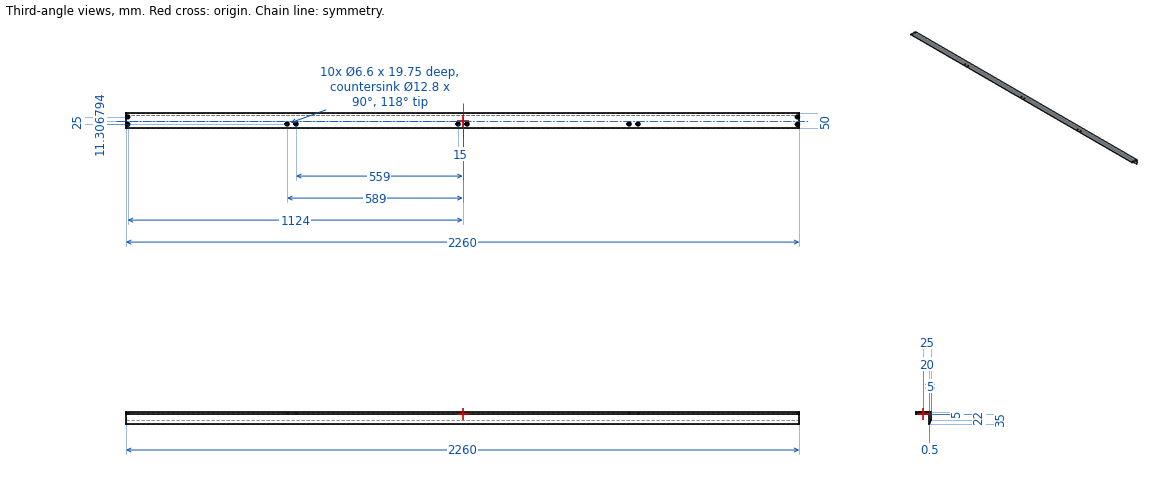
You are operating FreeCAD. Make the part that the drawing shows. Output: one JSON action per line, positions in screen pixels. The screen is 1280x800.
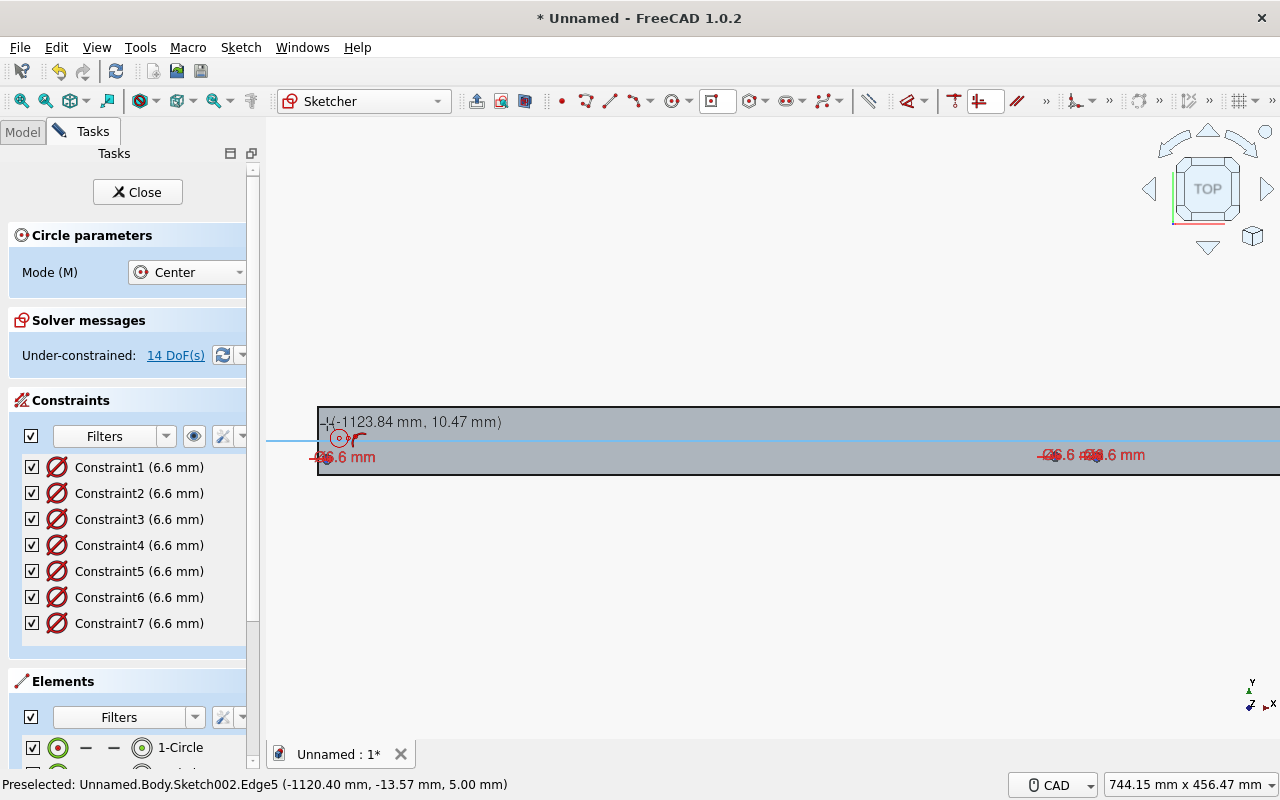
{"action": "left_click", "coordinate": [327, 424]}
{"action": "mouse_move", "coordinate": [330, 421]}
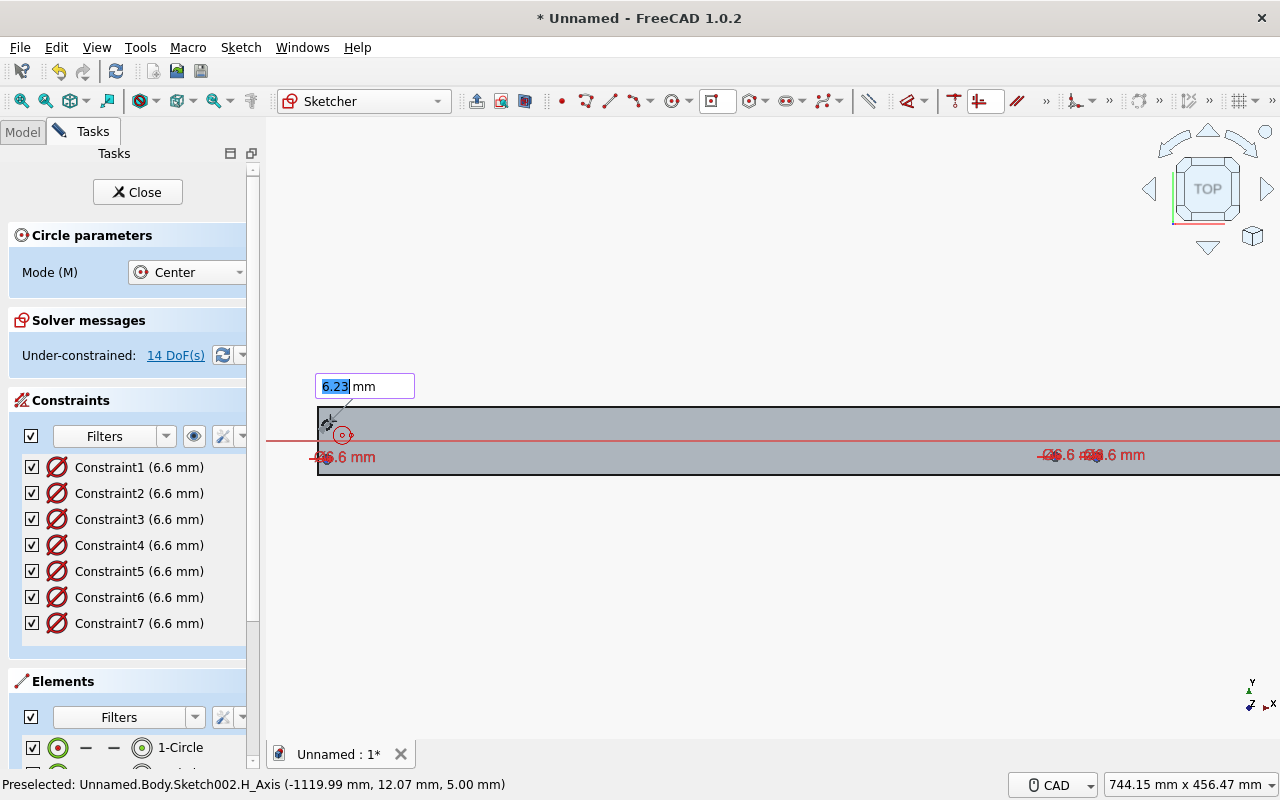
{"action": "type", "text": "6.6"}
{"action": "key", "text": "Return"}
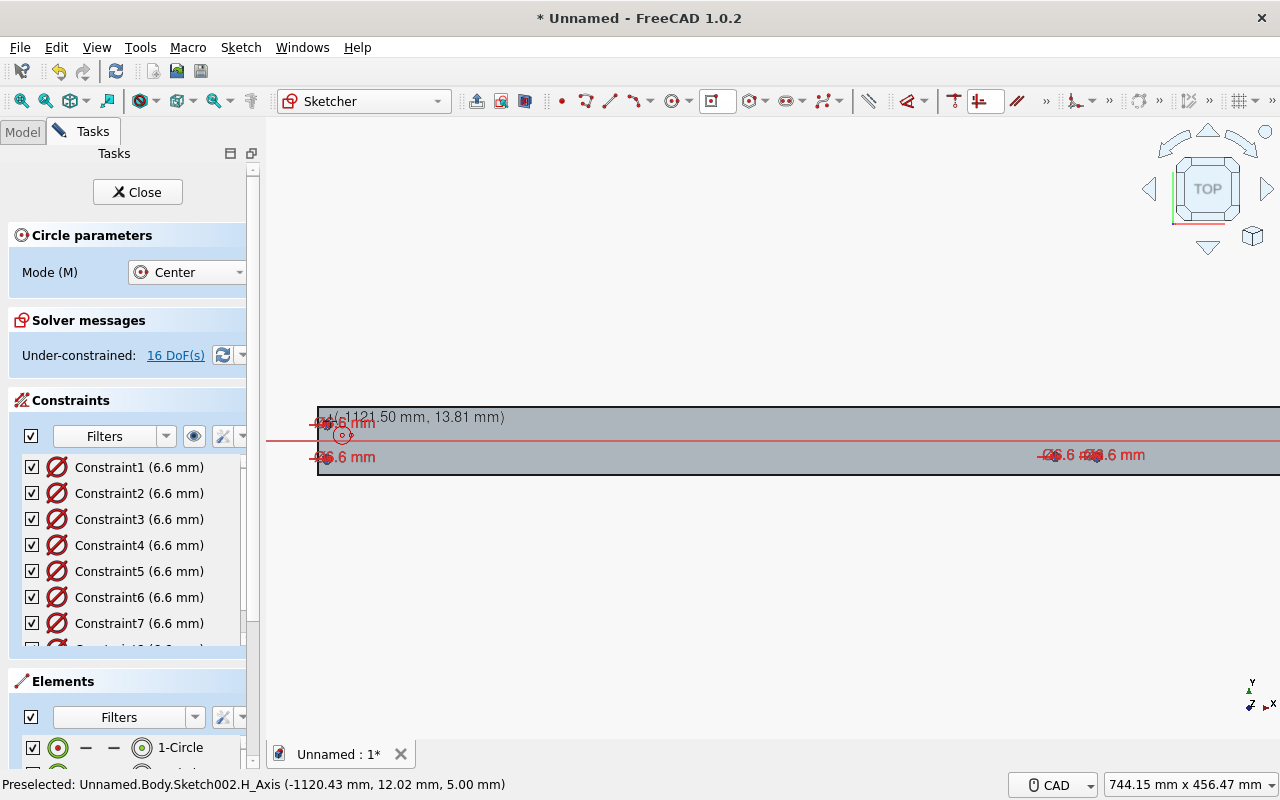
{"action": "scroll", "coordinate": [413, 425], "scroll_direction": "down", "scroll_amount": 8}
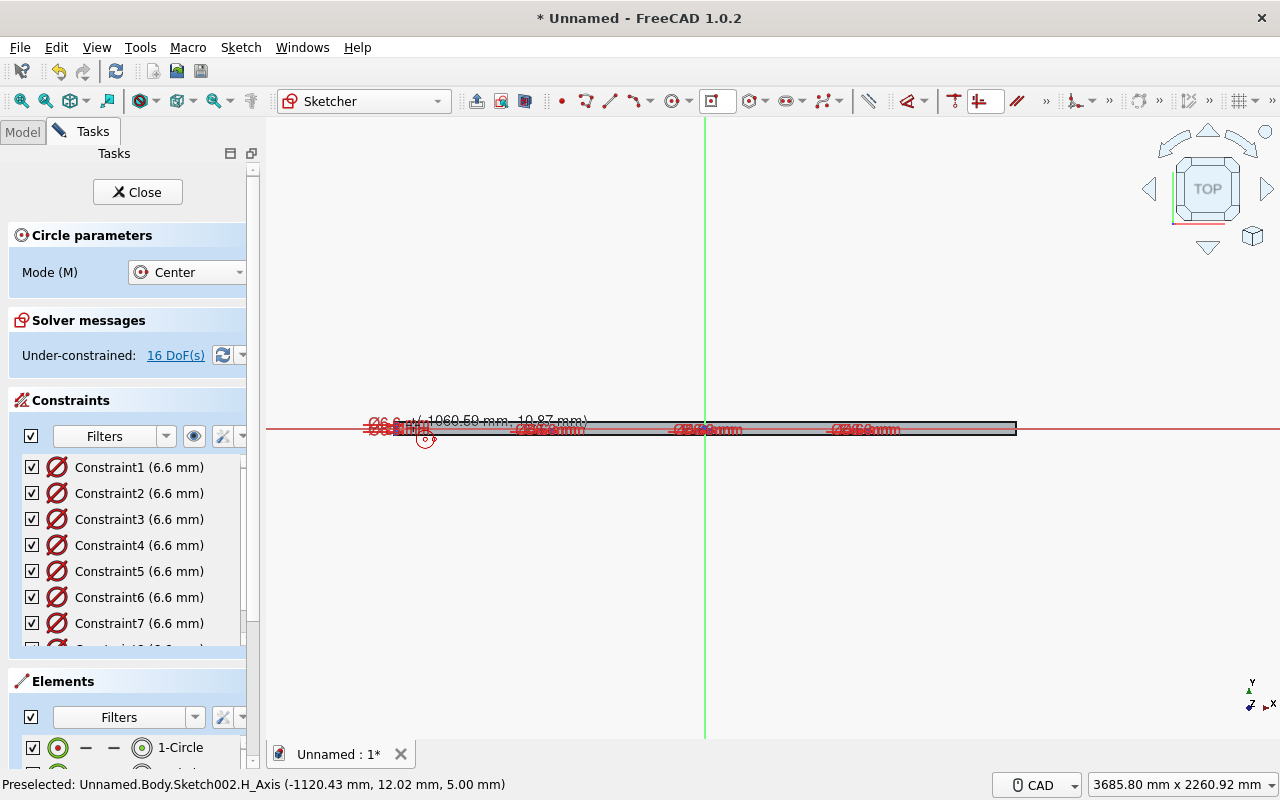
{"action": "scroll", "coordinate": [1014, 432], "scroll_direction": "up", "scroll_amount": 17}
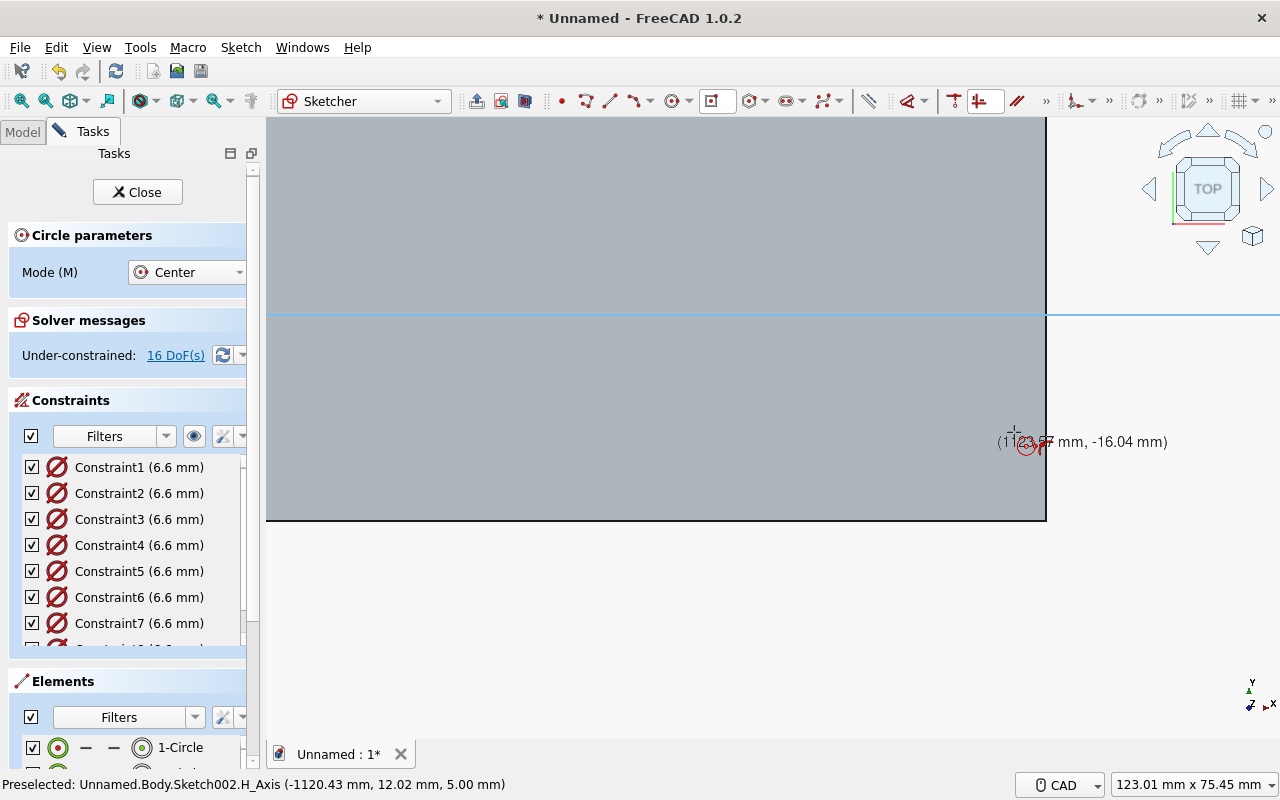
{"action": "scroll", "coordinate": [1086, 433], "scroll_direction": "down", "scroll_amount": 16}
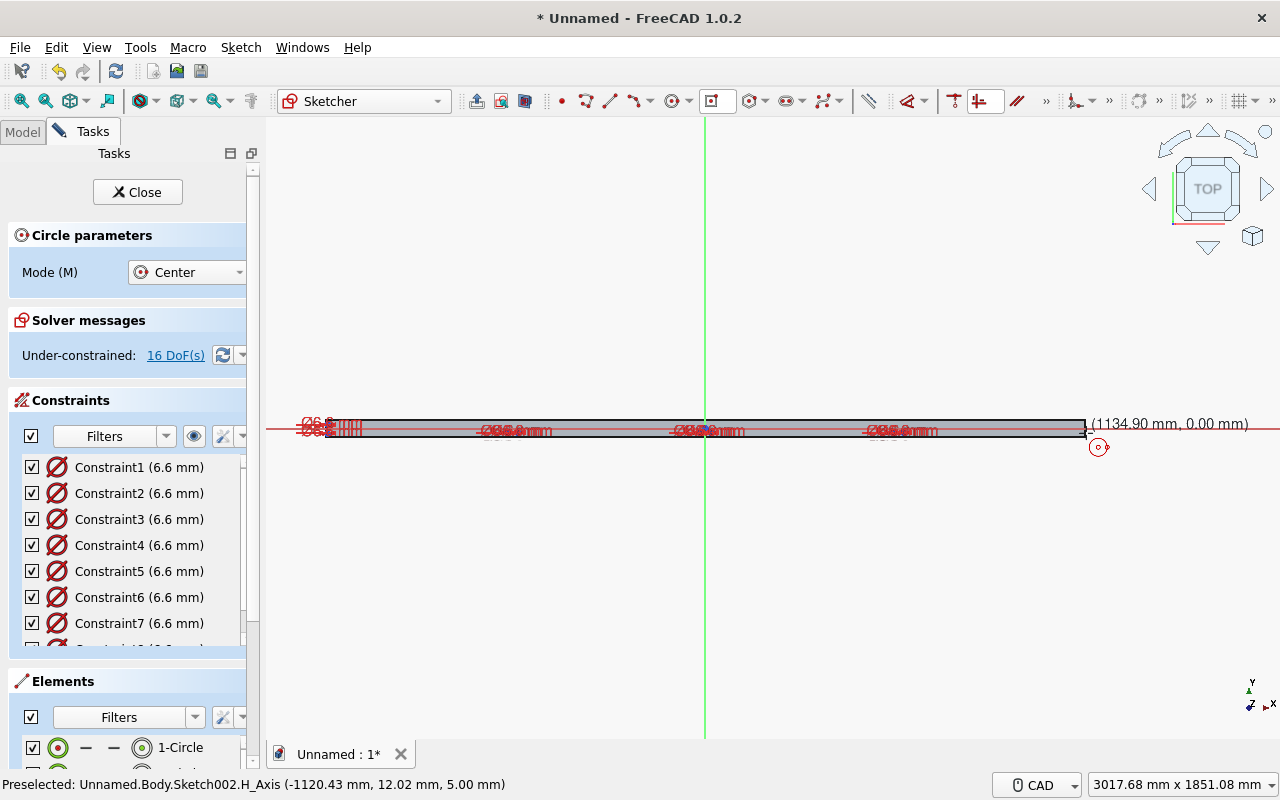
{"action": "scroll", "coordinate": [1083, 433], "scroll_direction": "up", "scroll_amount": 7}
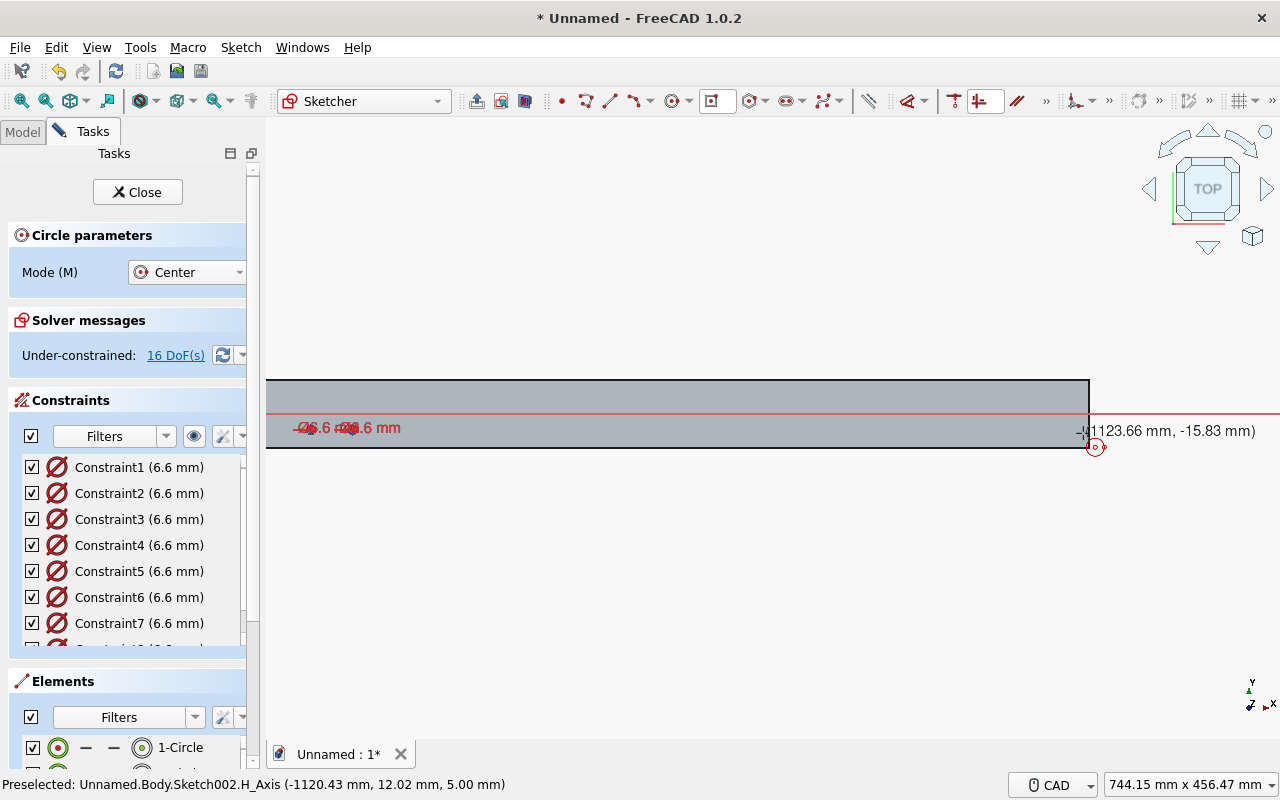
{"action": "left_click", "coordinate": [1081, 431]}
{"action": "mouse_move", "coordinate": [1084, 434]}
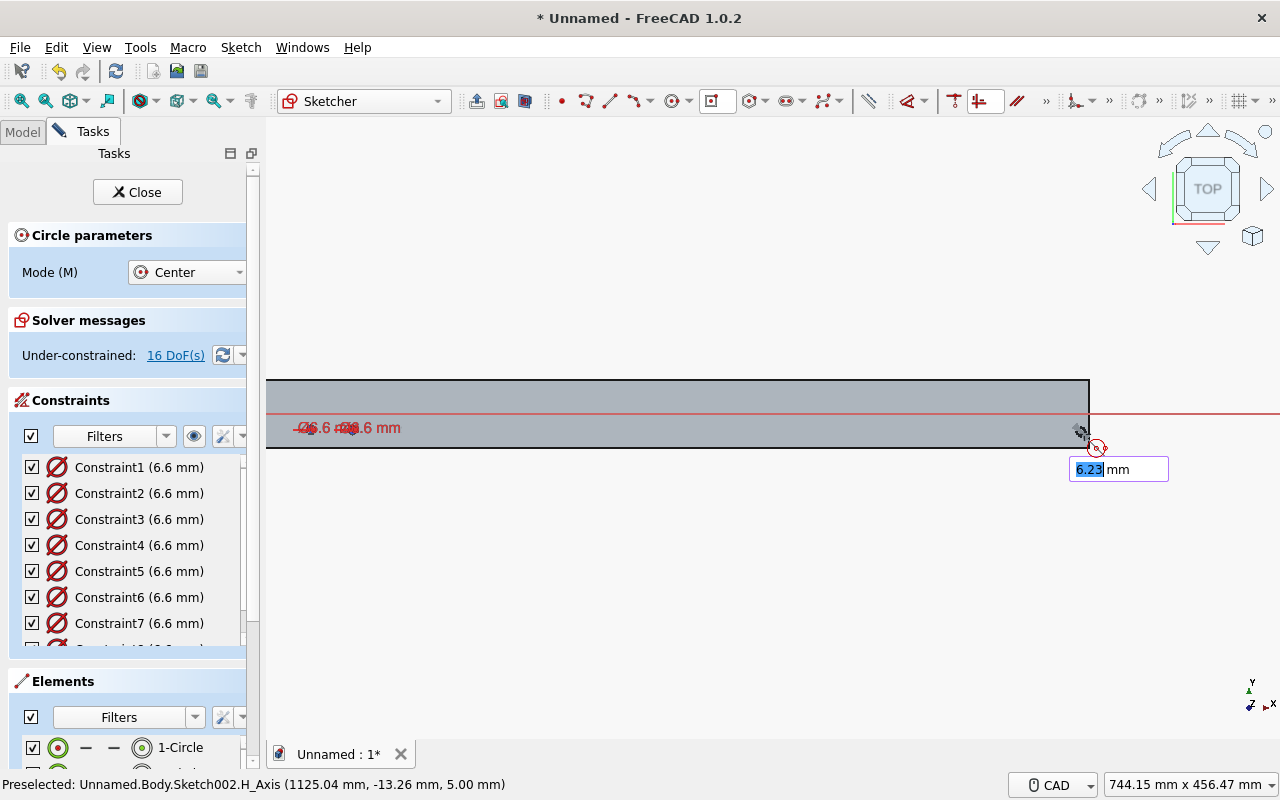
{"action": "type", "text": "6.6"}
{"action": "key", "text": "Return"}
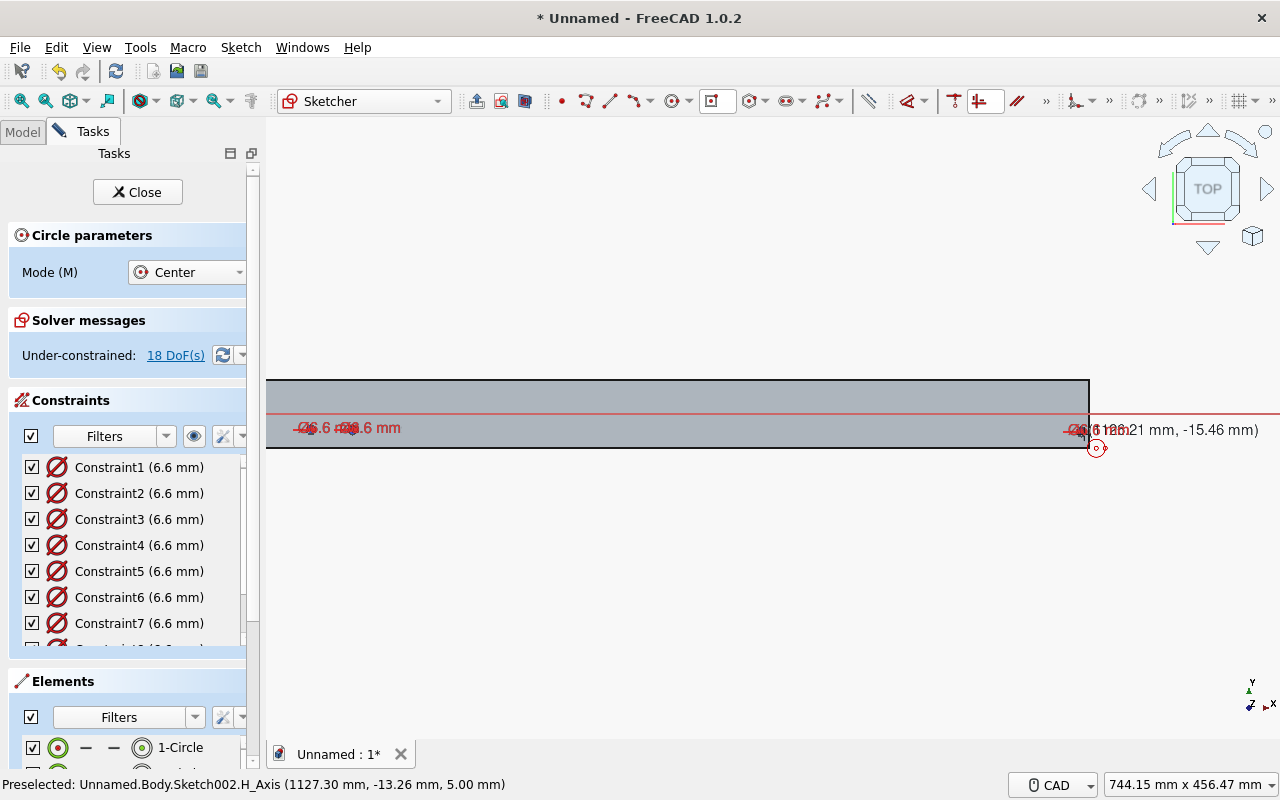
{"action": "scroll", "coordinate": [1081, 397], "scroll_direction": "up", "scroll_amount": 9}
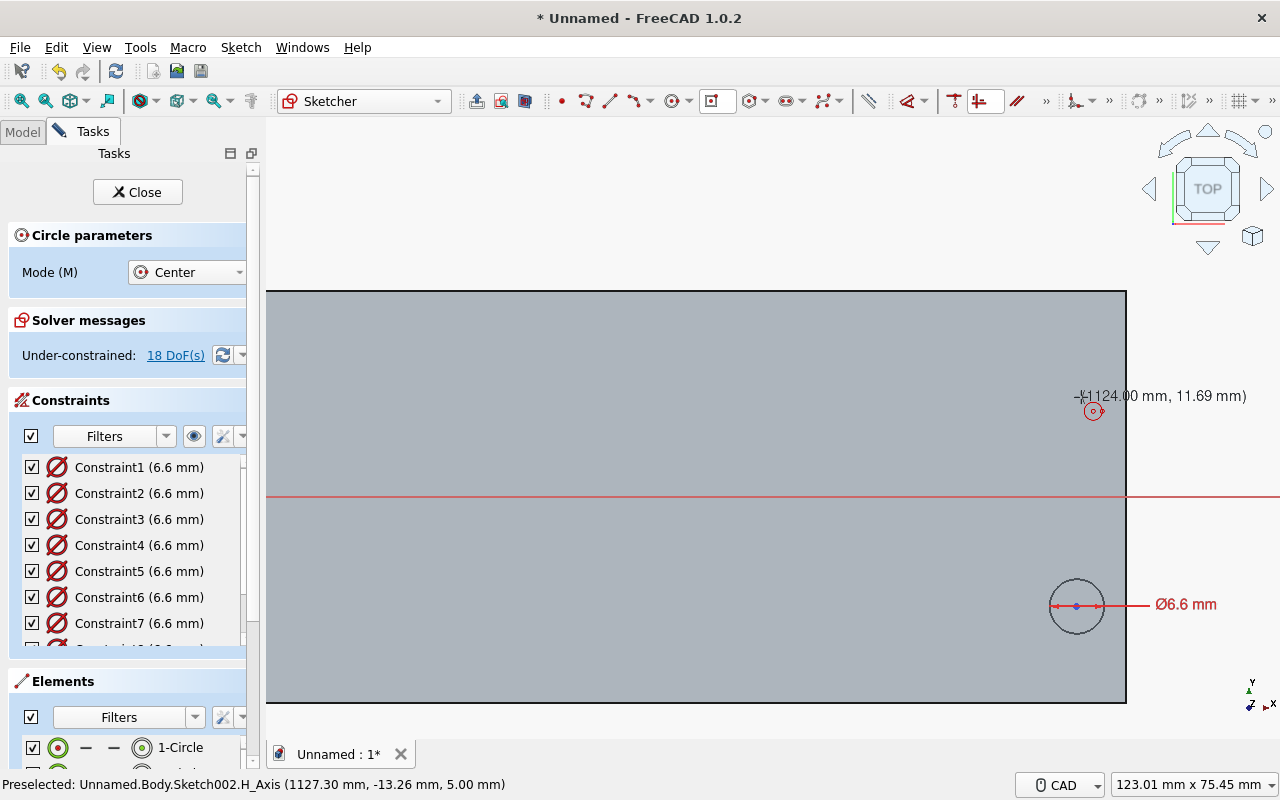
{"action": "scroll", "coordinate": [1082, 425], "scroll_direction": "down", "scroll_amount": 16}